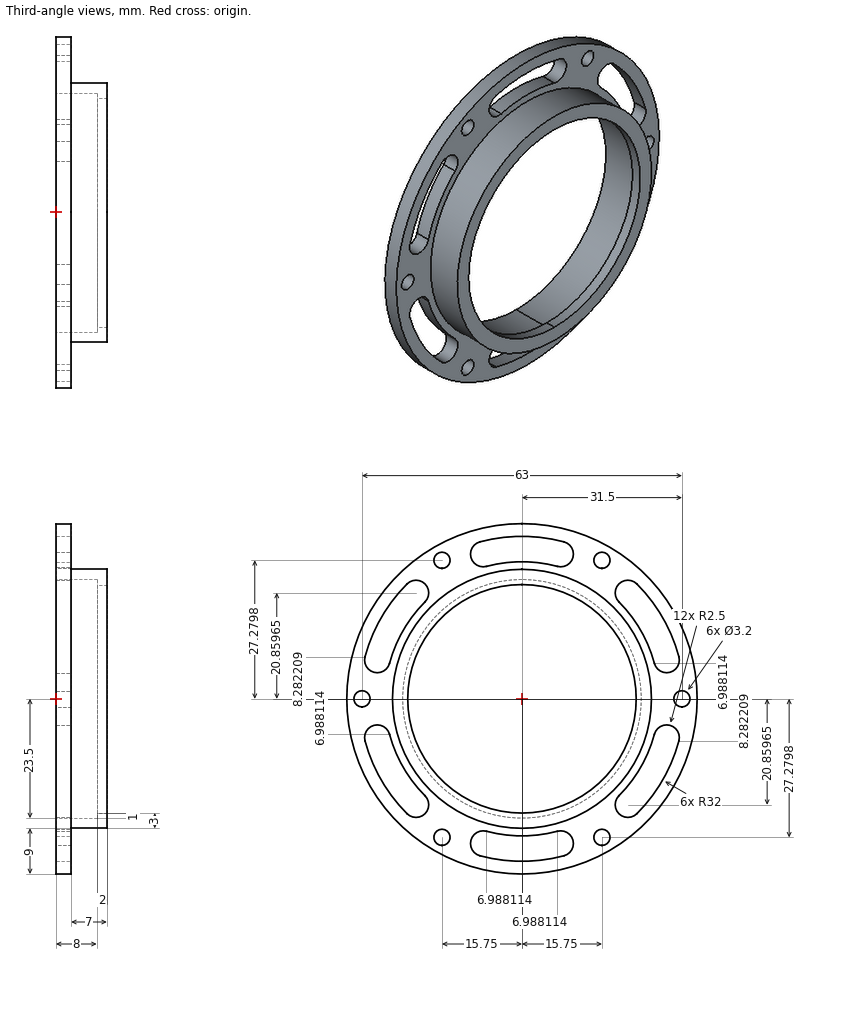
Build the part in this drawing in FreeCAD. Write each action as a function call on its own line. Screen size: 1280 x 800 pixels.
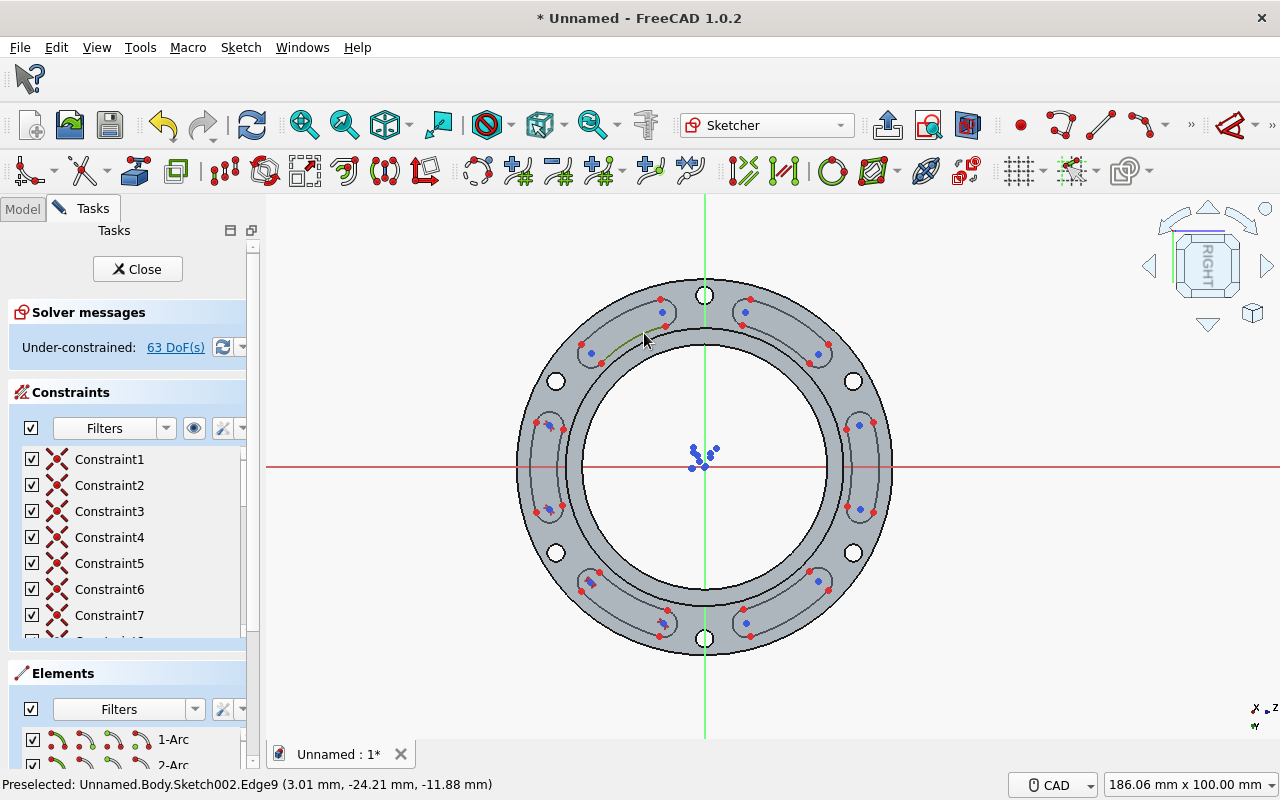
click(578, 357)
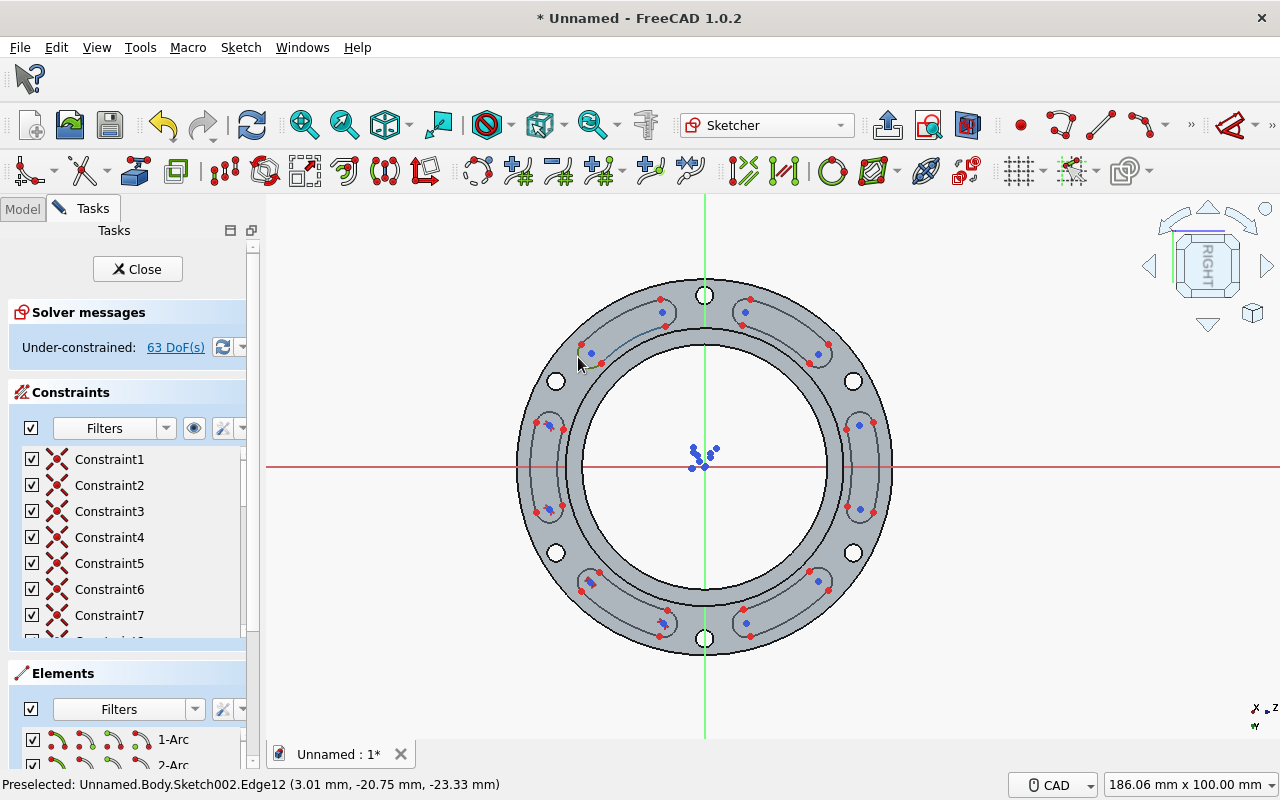
key(t)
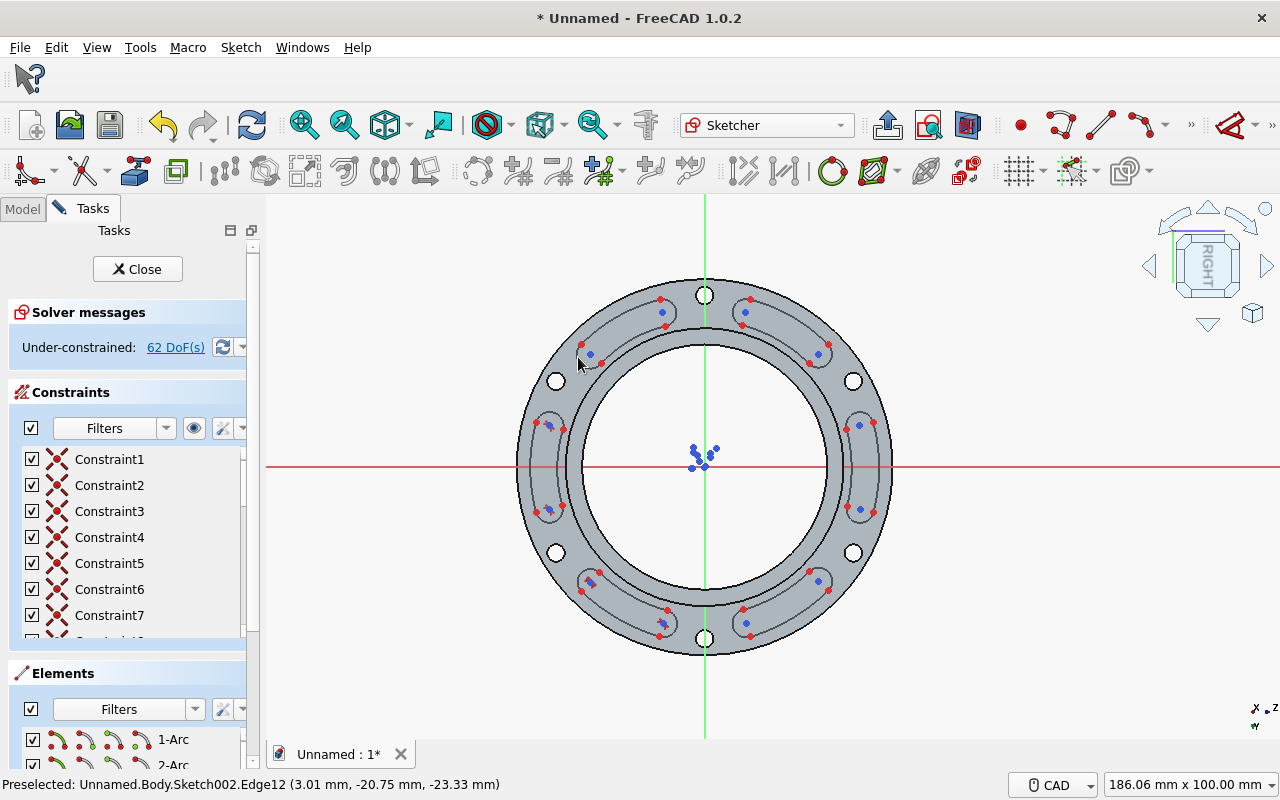
click(675, 318)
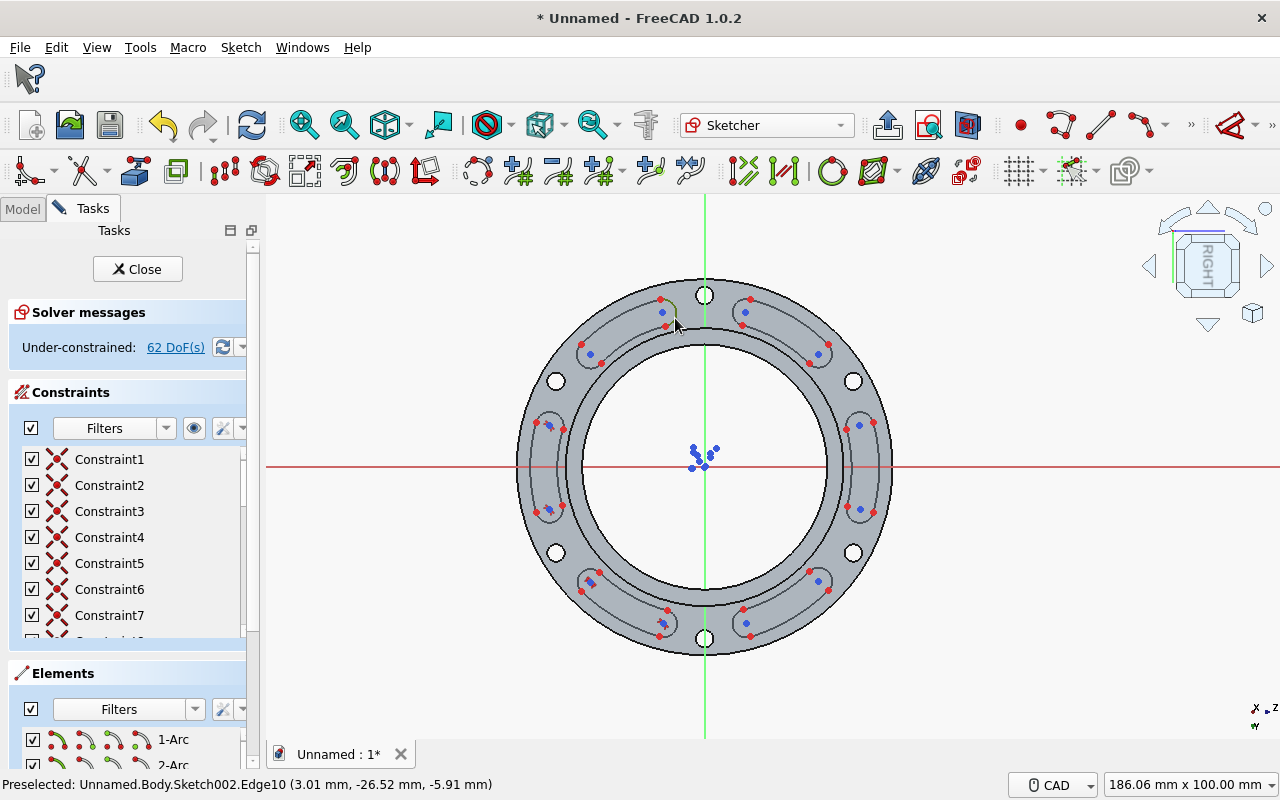
click(634, 308)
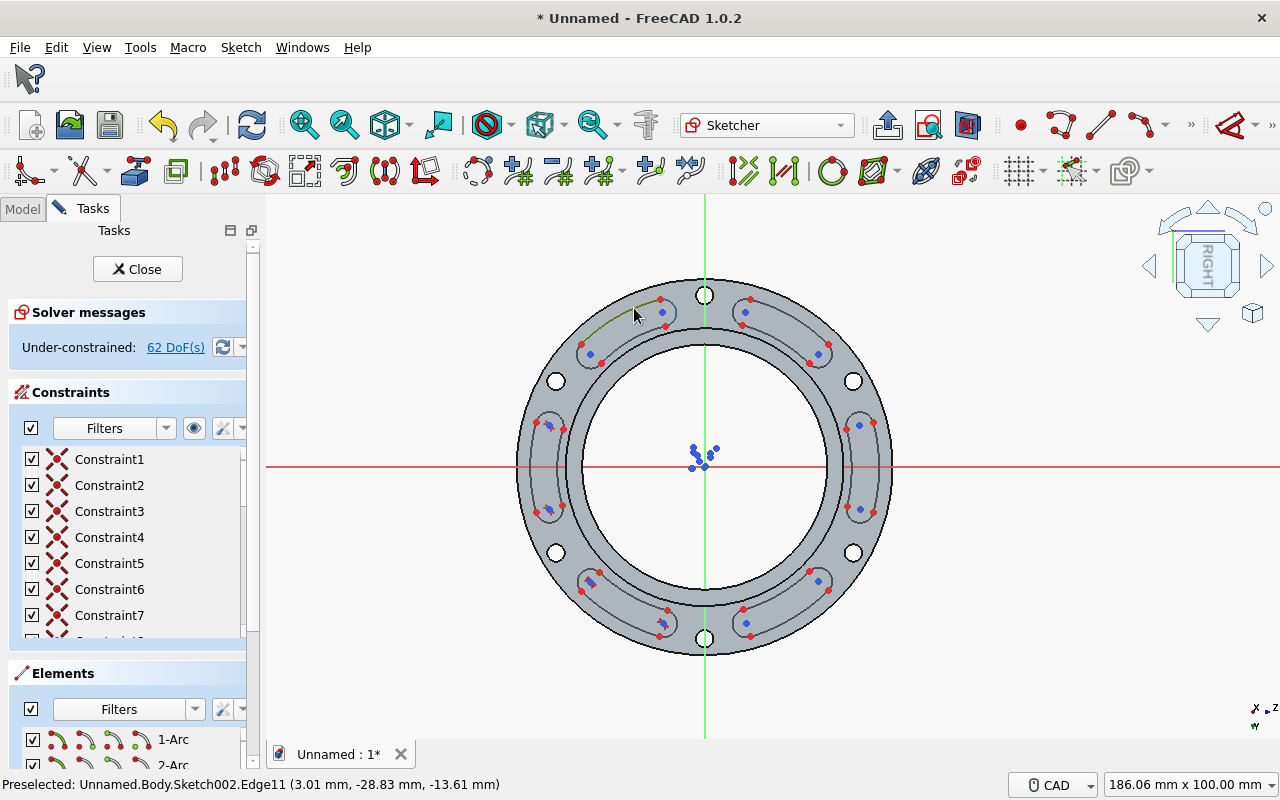
key(t)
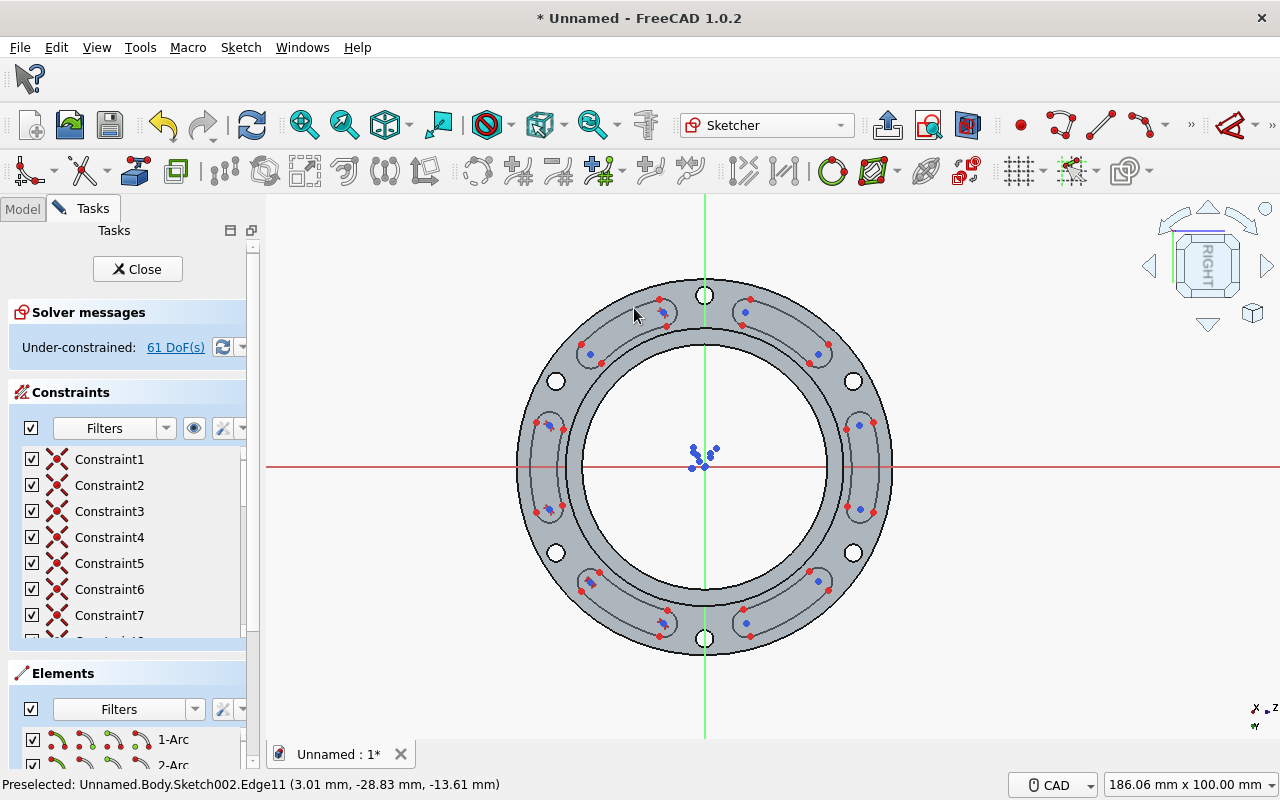
click(634, 308)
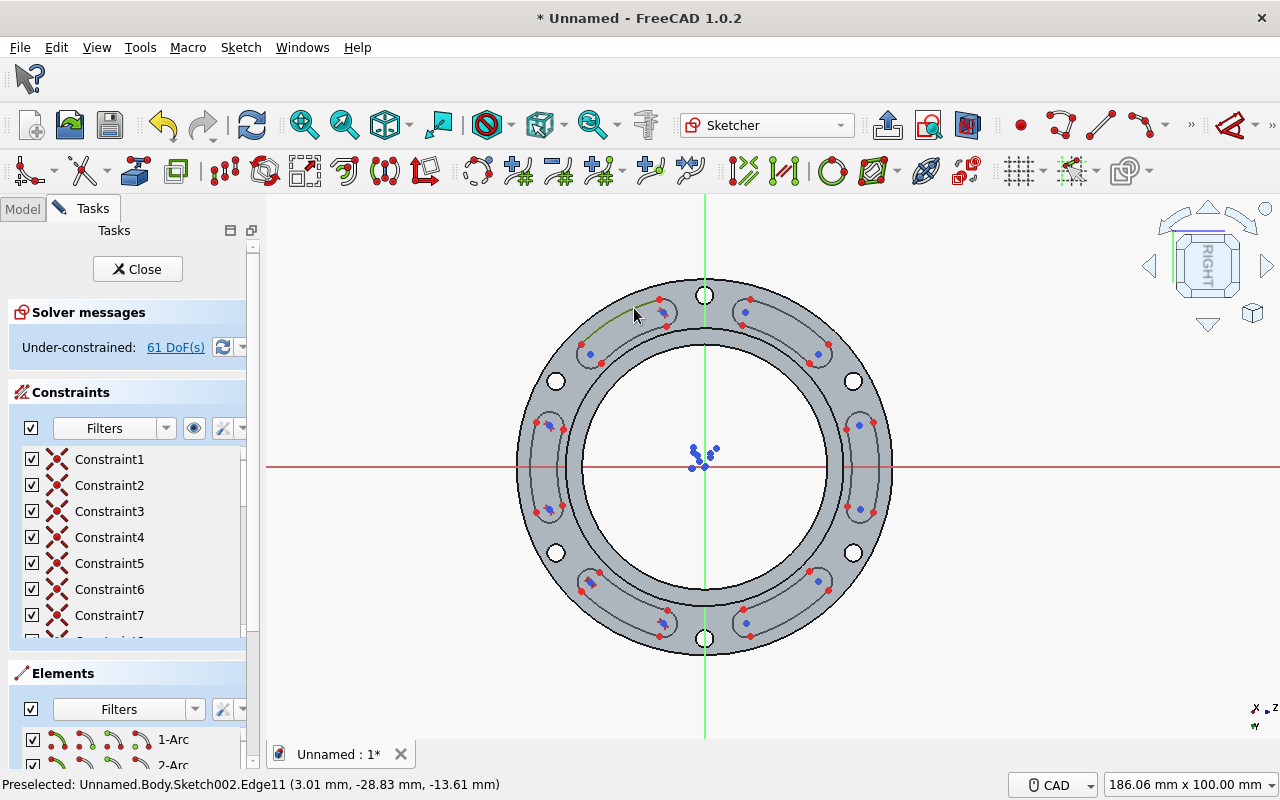
click(577, 357)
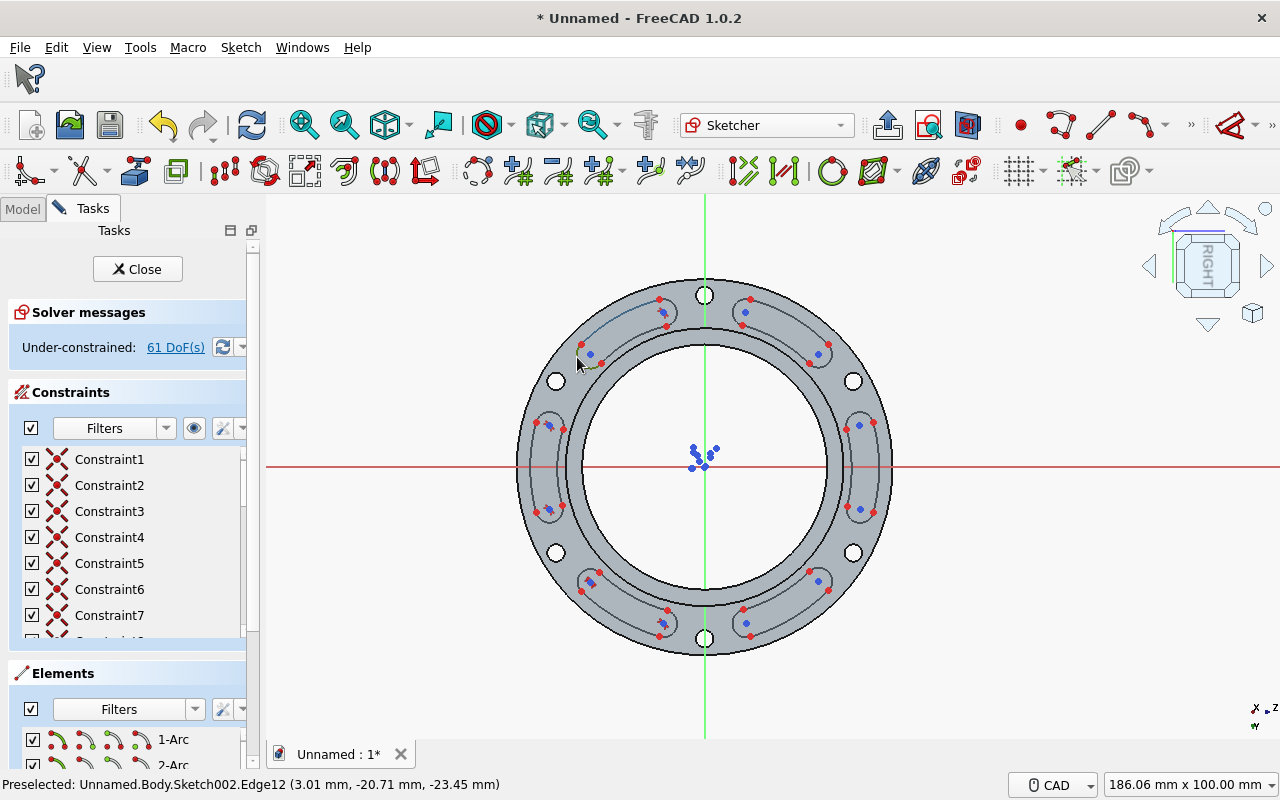
key(t)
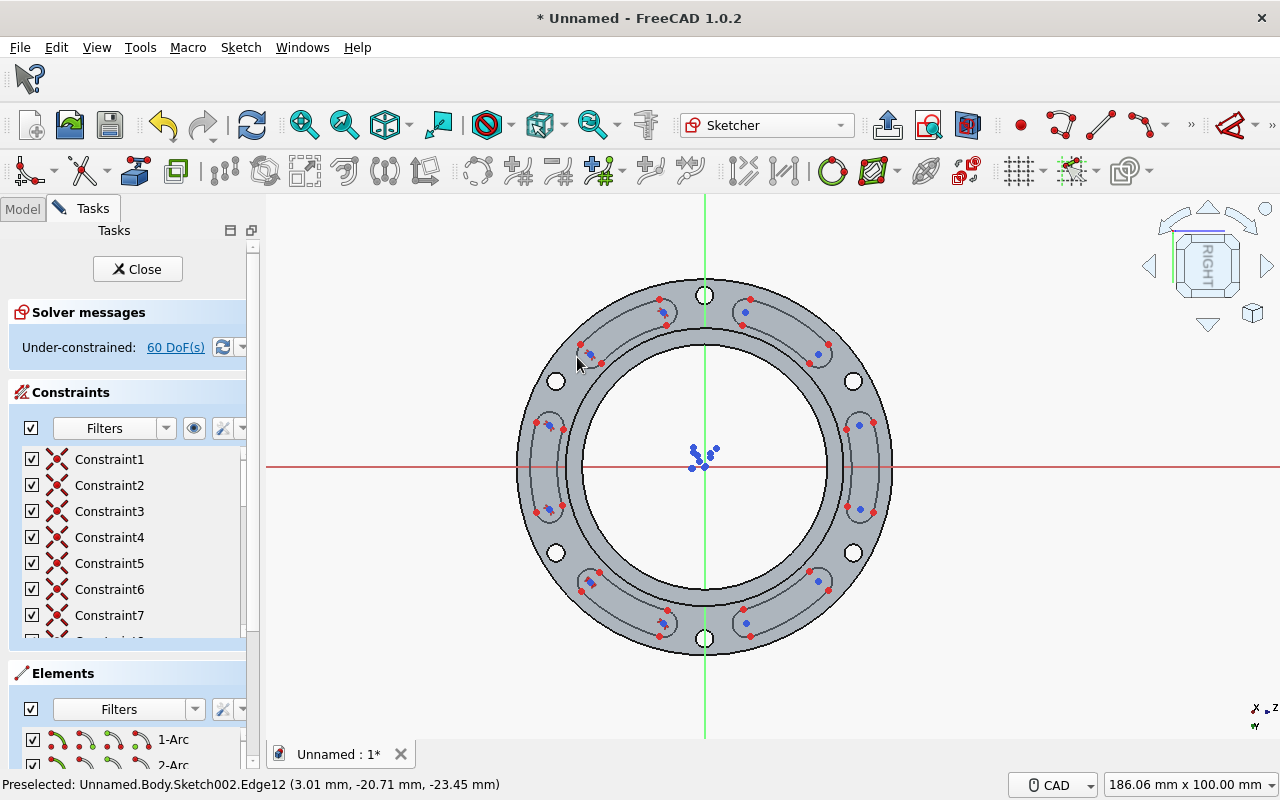
click(821, 367)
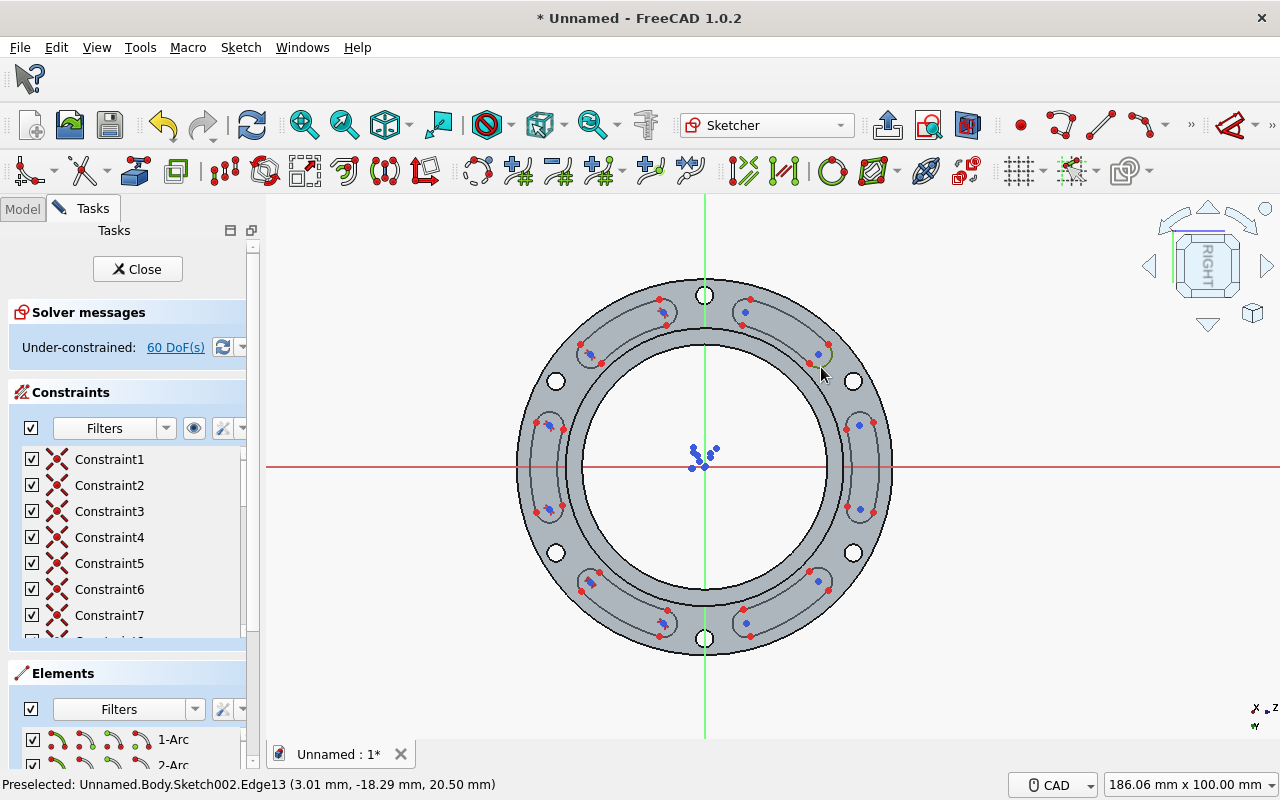
click(807, 327)